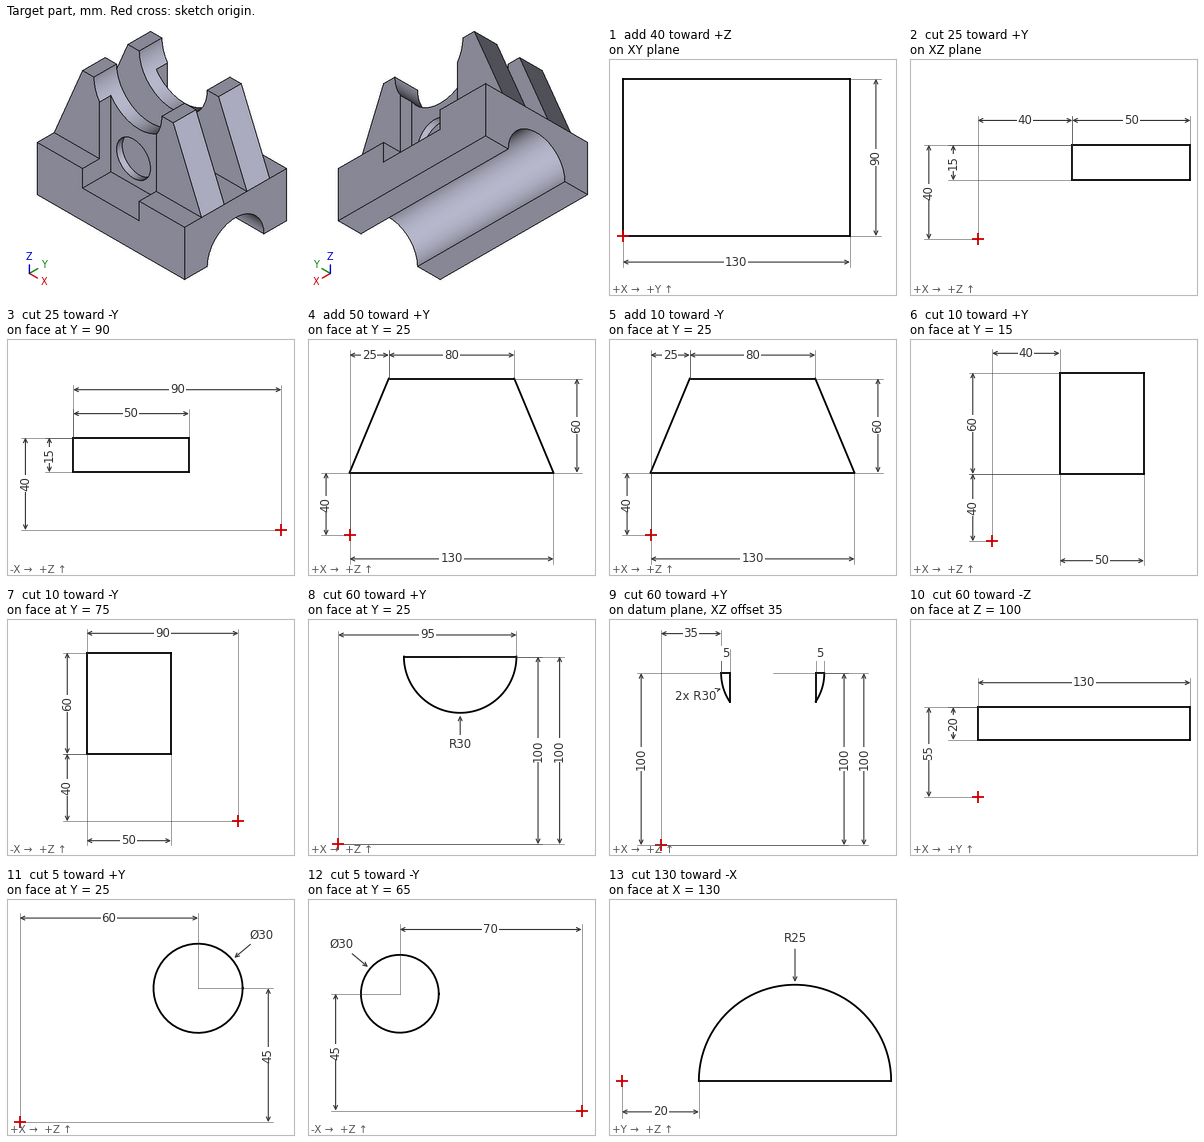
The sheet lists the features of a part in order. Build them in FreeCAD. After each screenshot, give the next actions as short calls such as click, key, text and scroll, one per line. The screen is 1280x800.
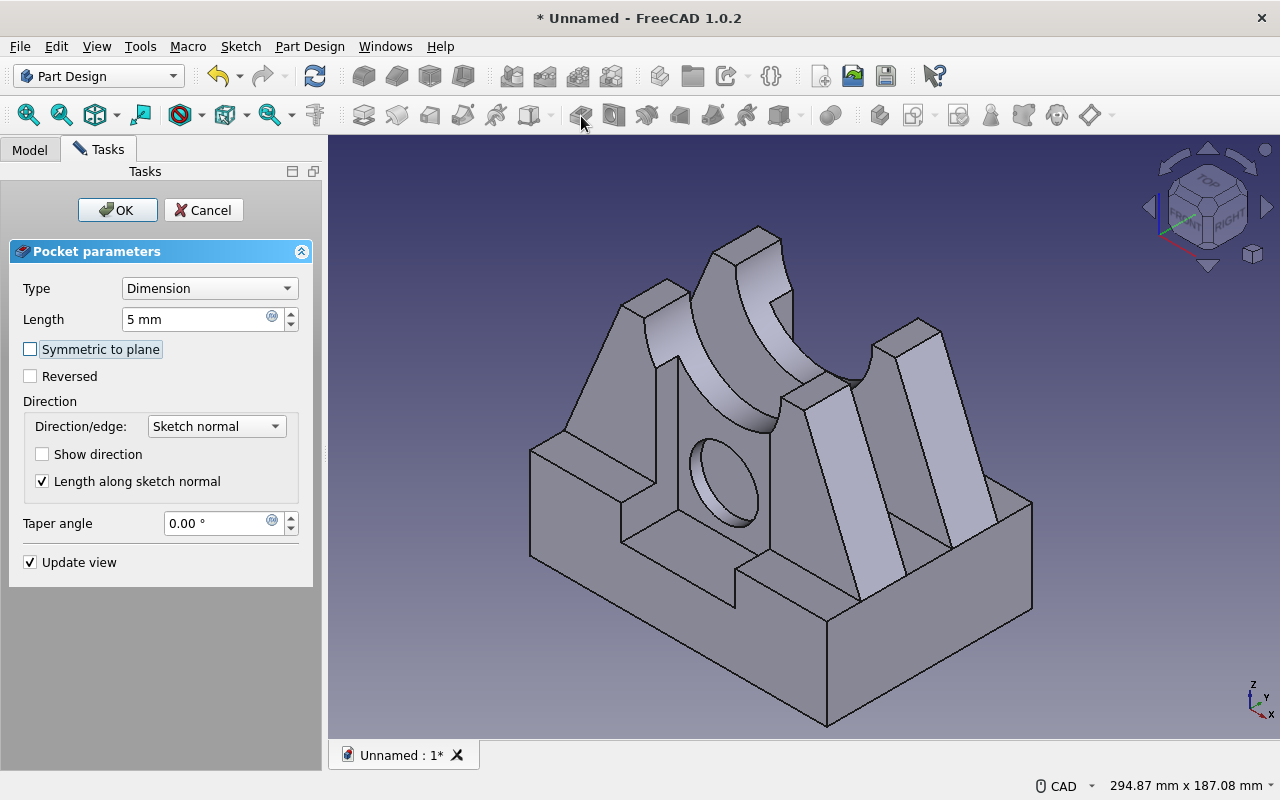
click(118, 210)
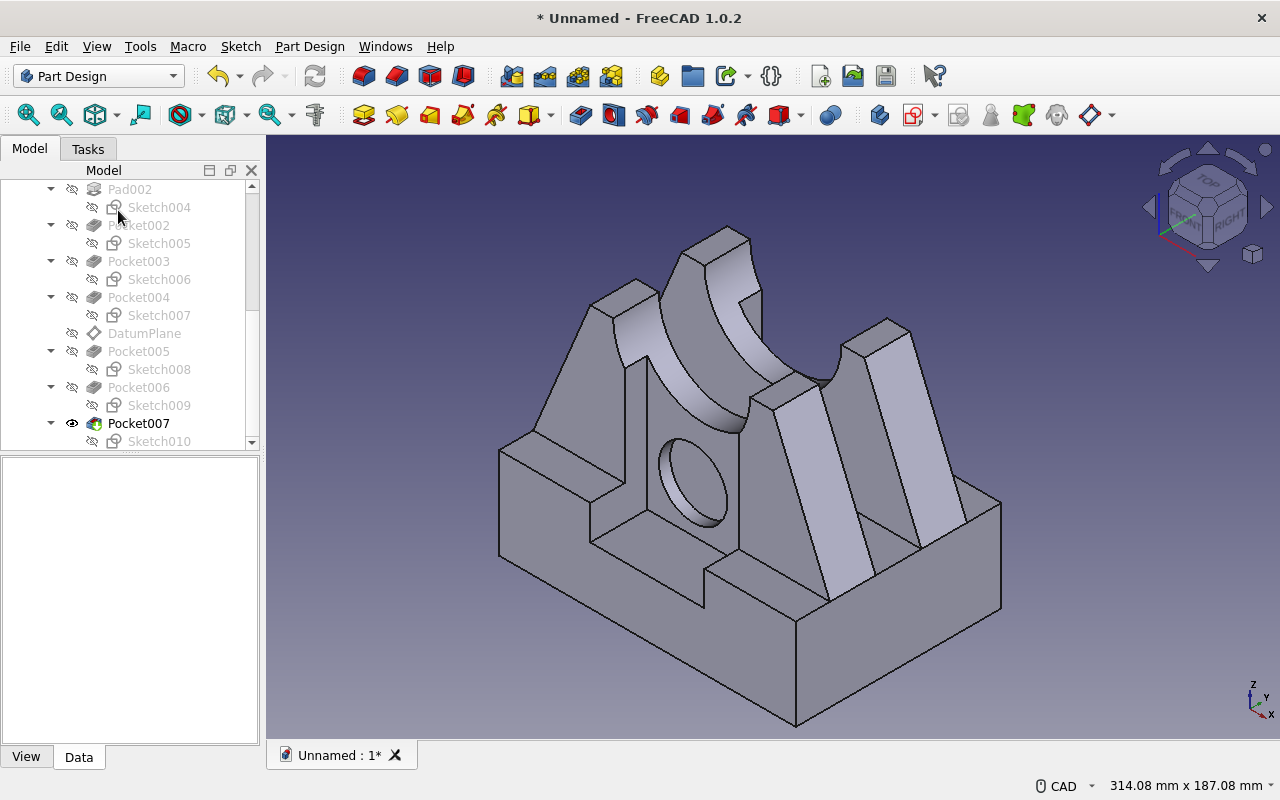
key(4)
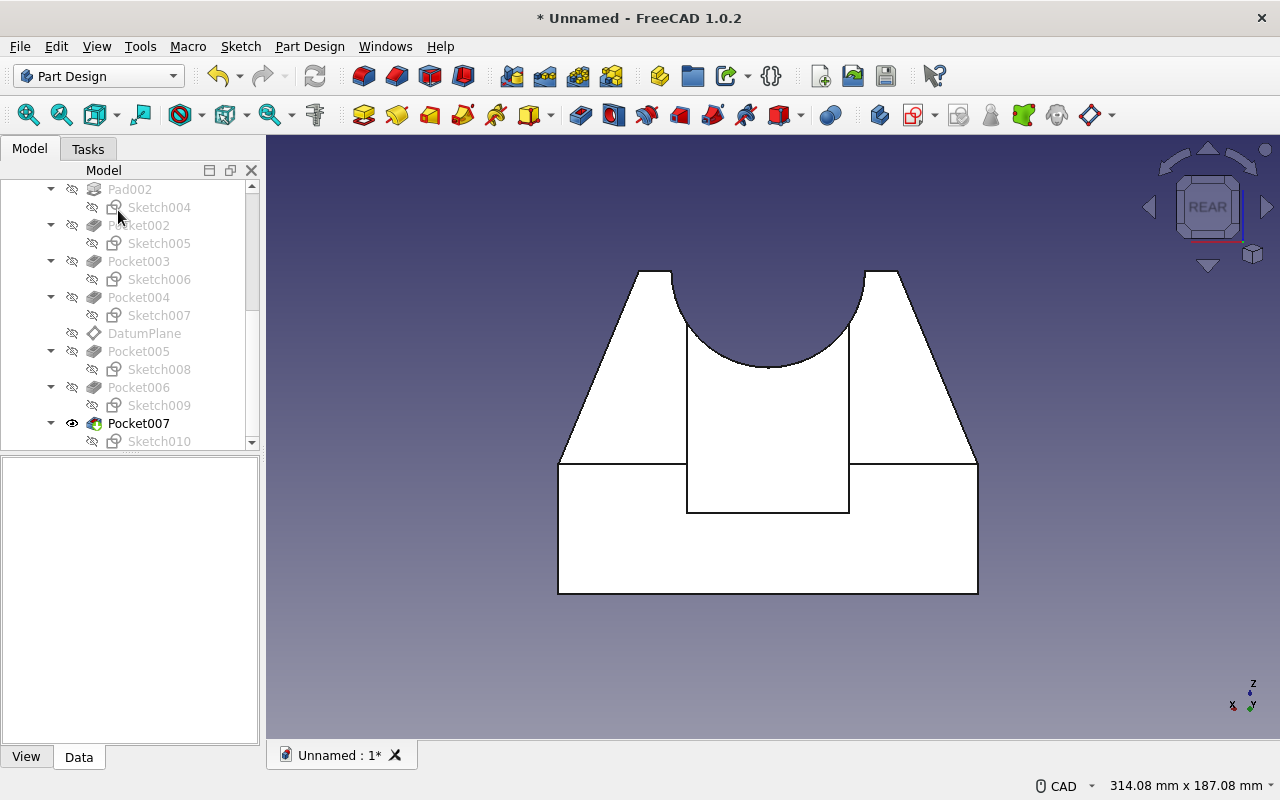
click(768, 445)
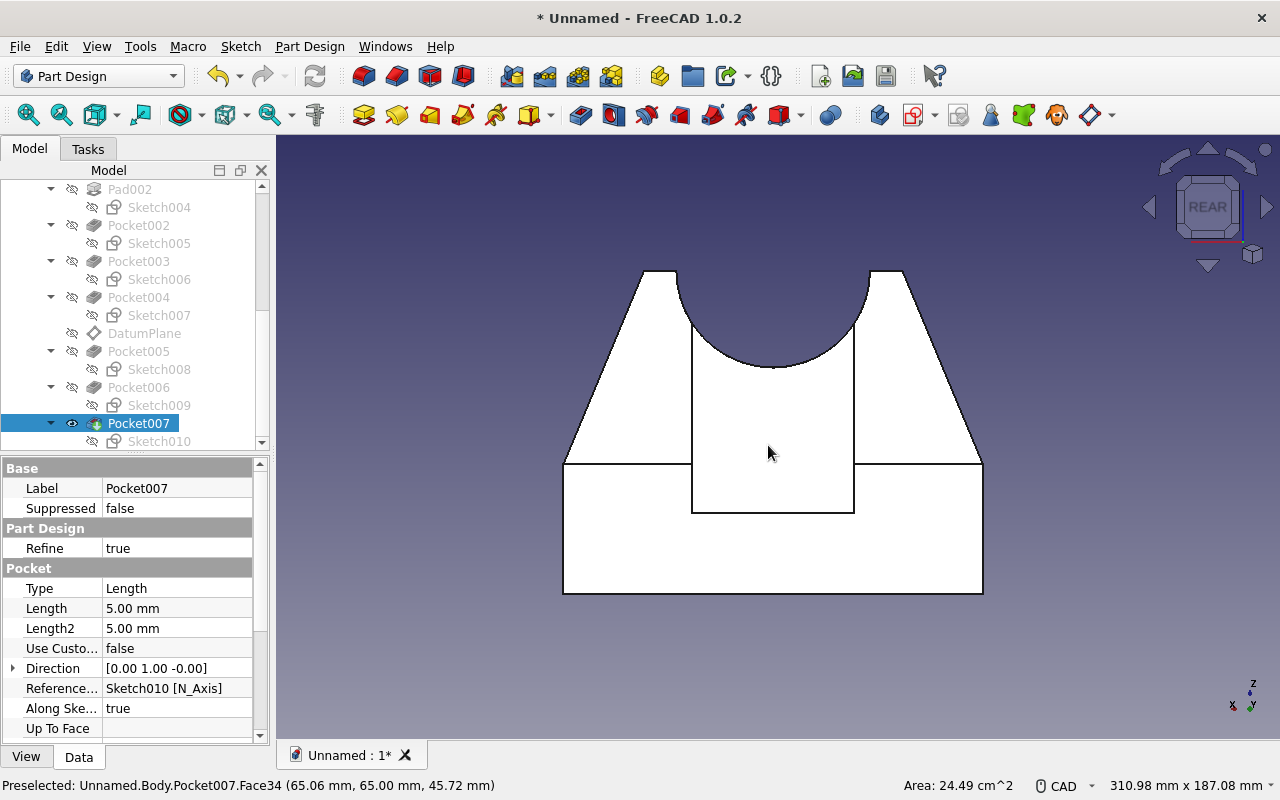
click(912, 116)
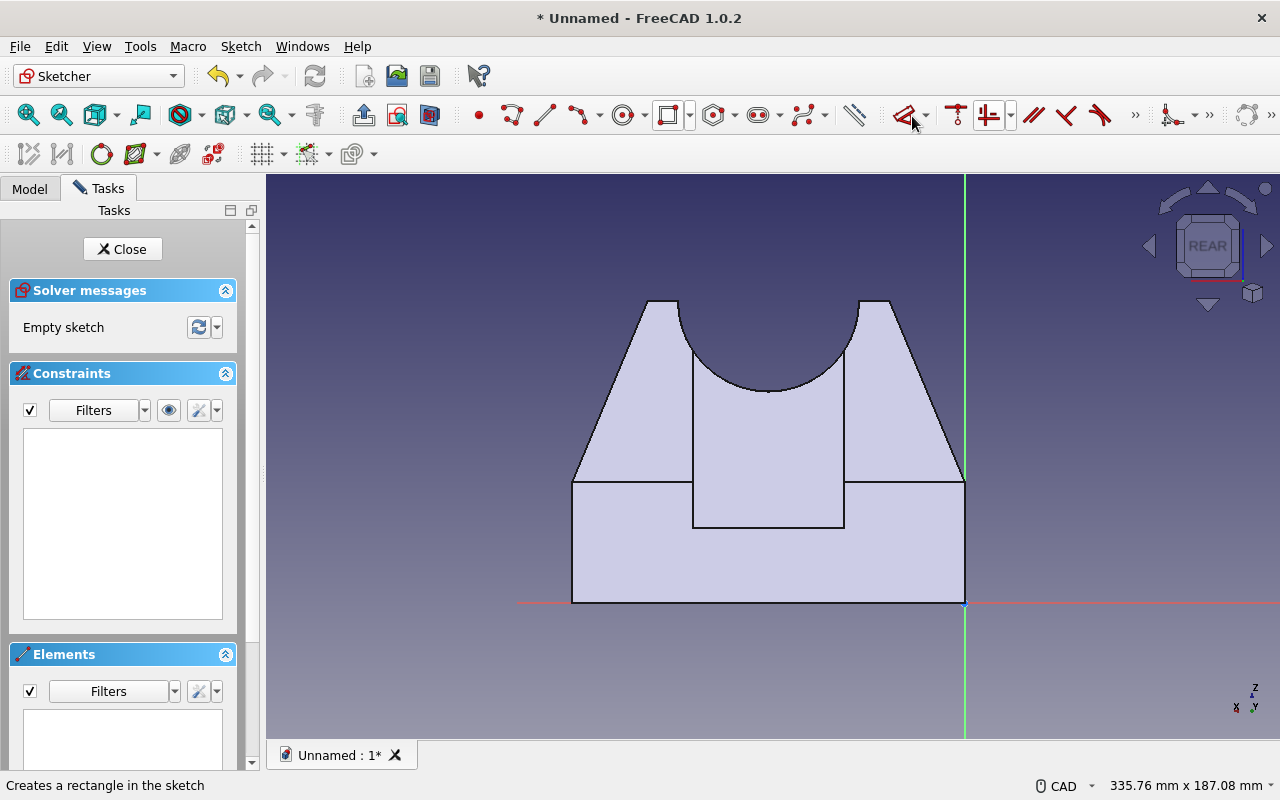
key(q)
key(s)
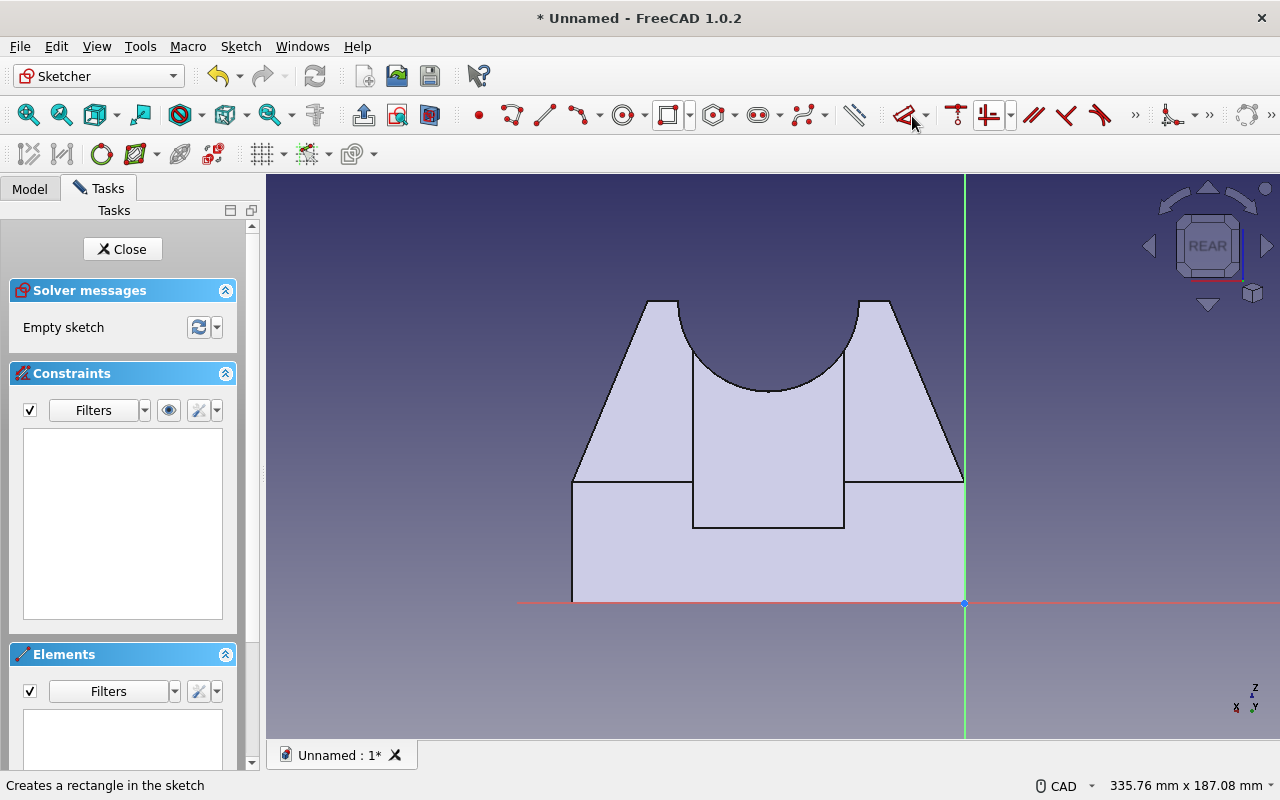
scroll(769, 471, up, 7)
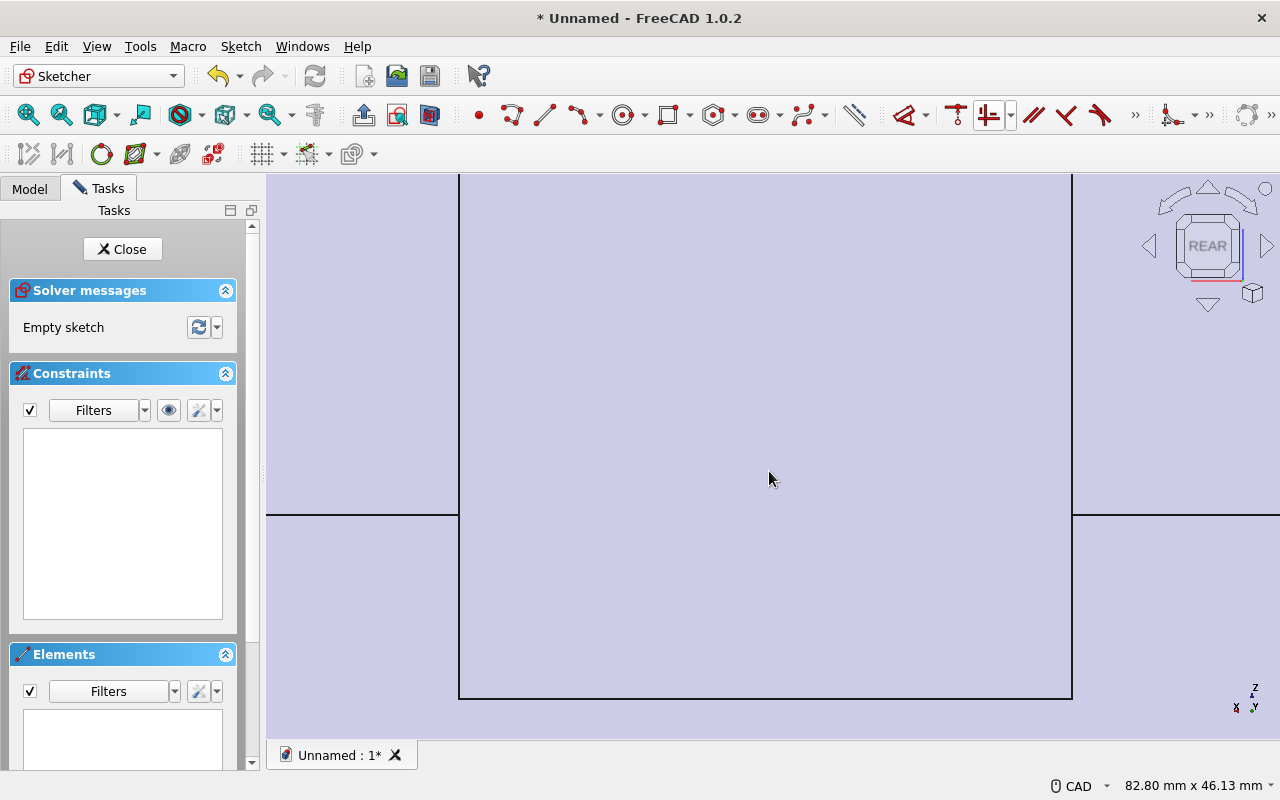
click(622, 116)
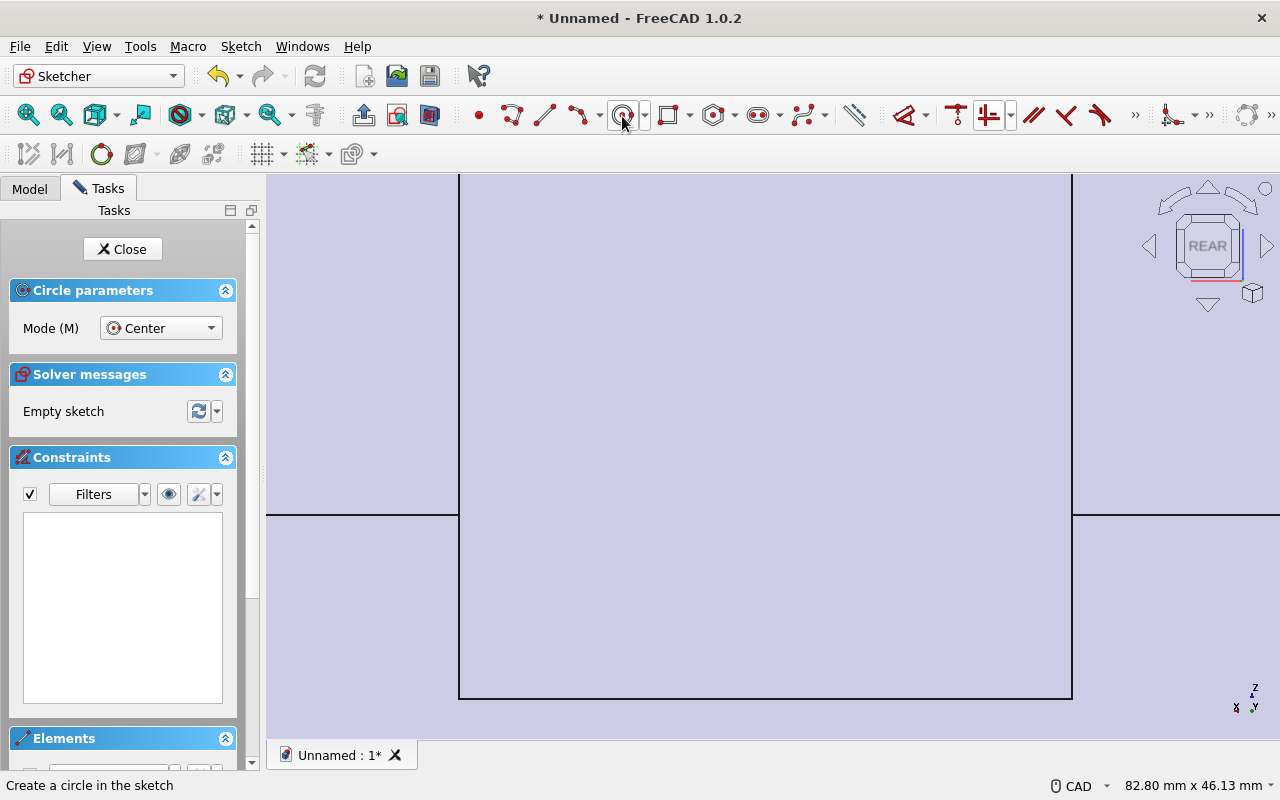
click(704, 454)
click(834, 324)
key(Escape)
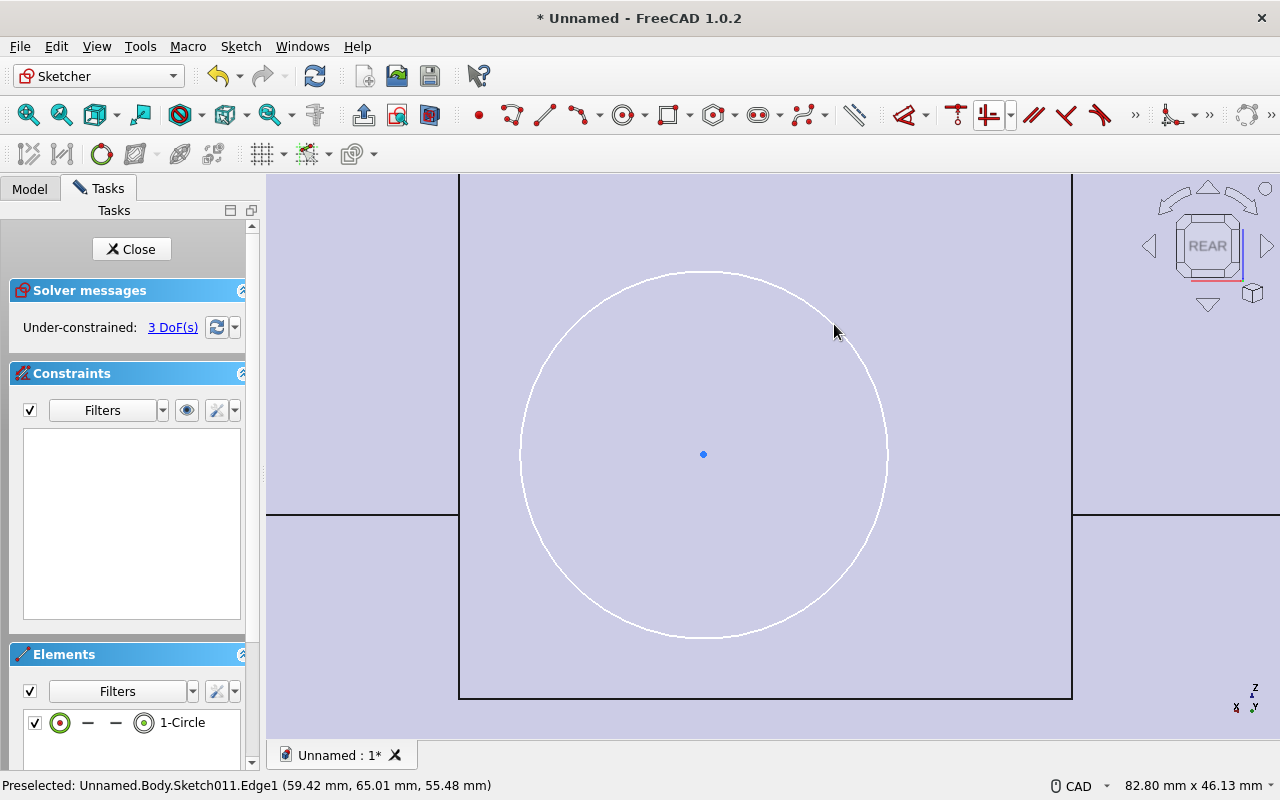
key(d)